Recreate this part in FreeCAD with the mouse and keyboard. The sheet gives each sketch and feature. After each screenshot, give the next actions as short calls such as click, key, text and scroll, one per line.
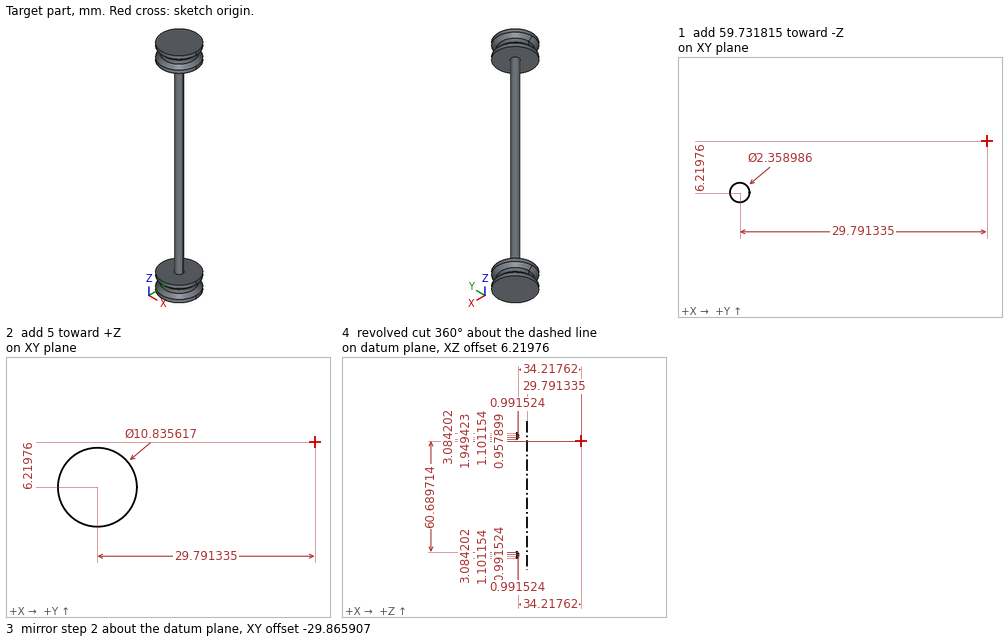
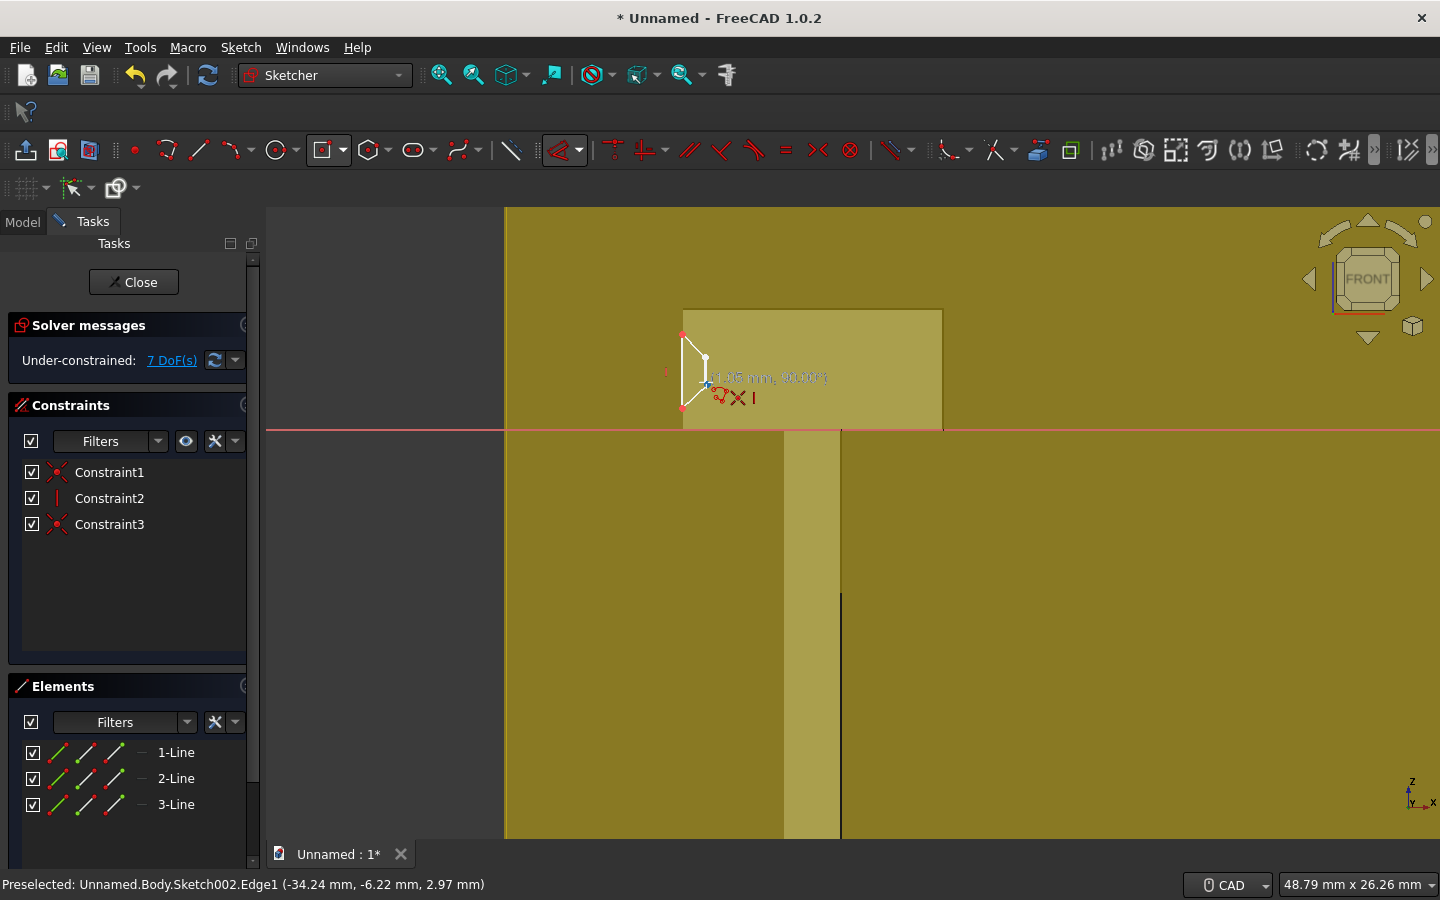
click(708, 385)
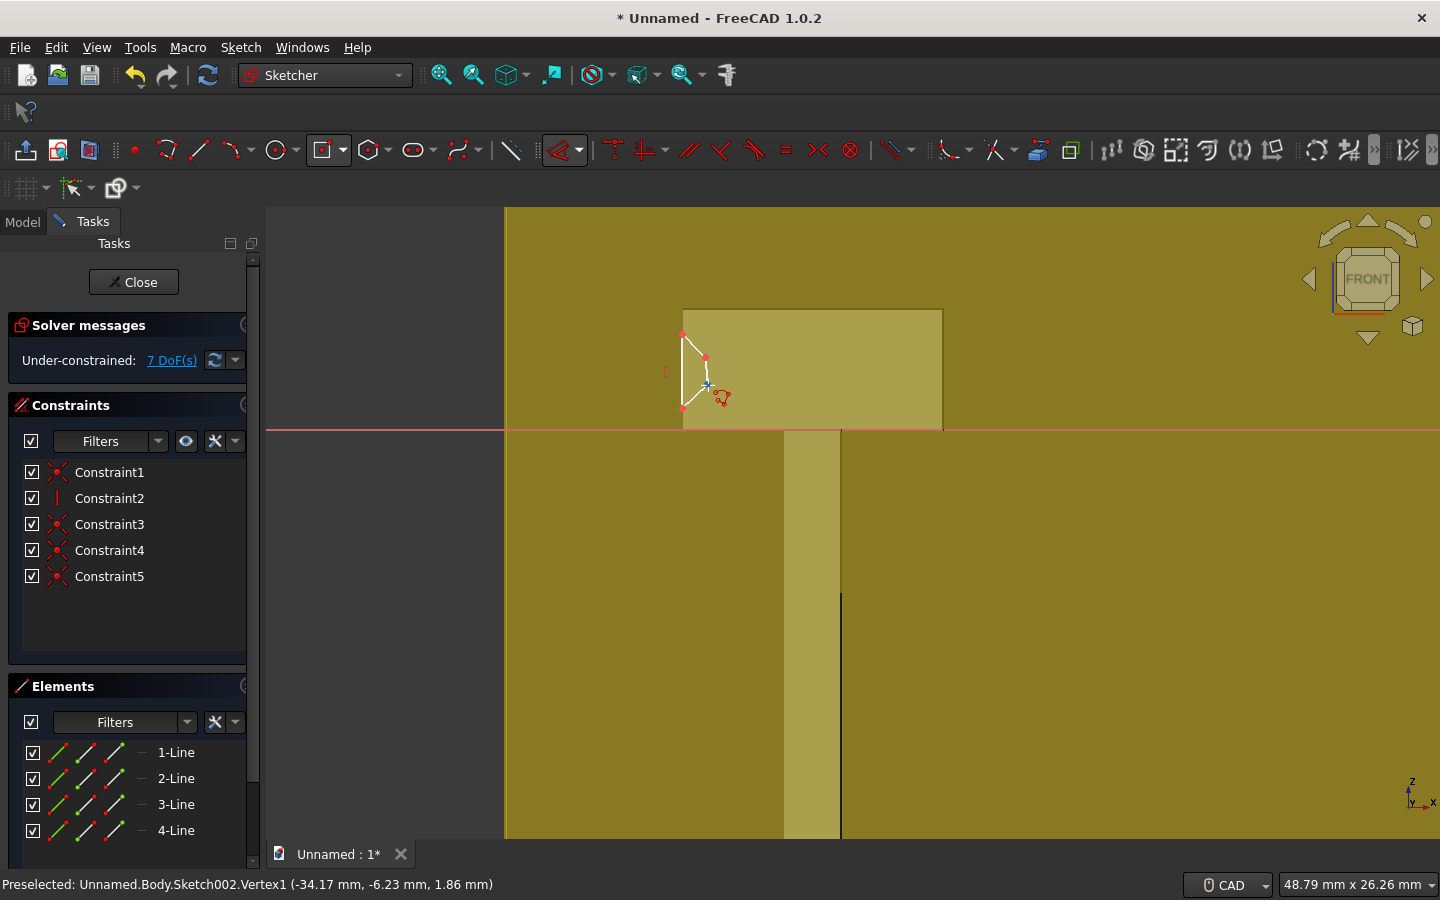
scroll(703, 365, down, 8)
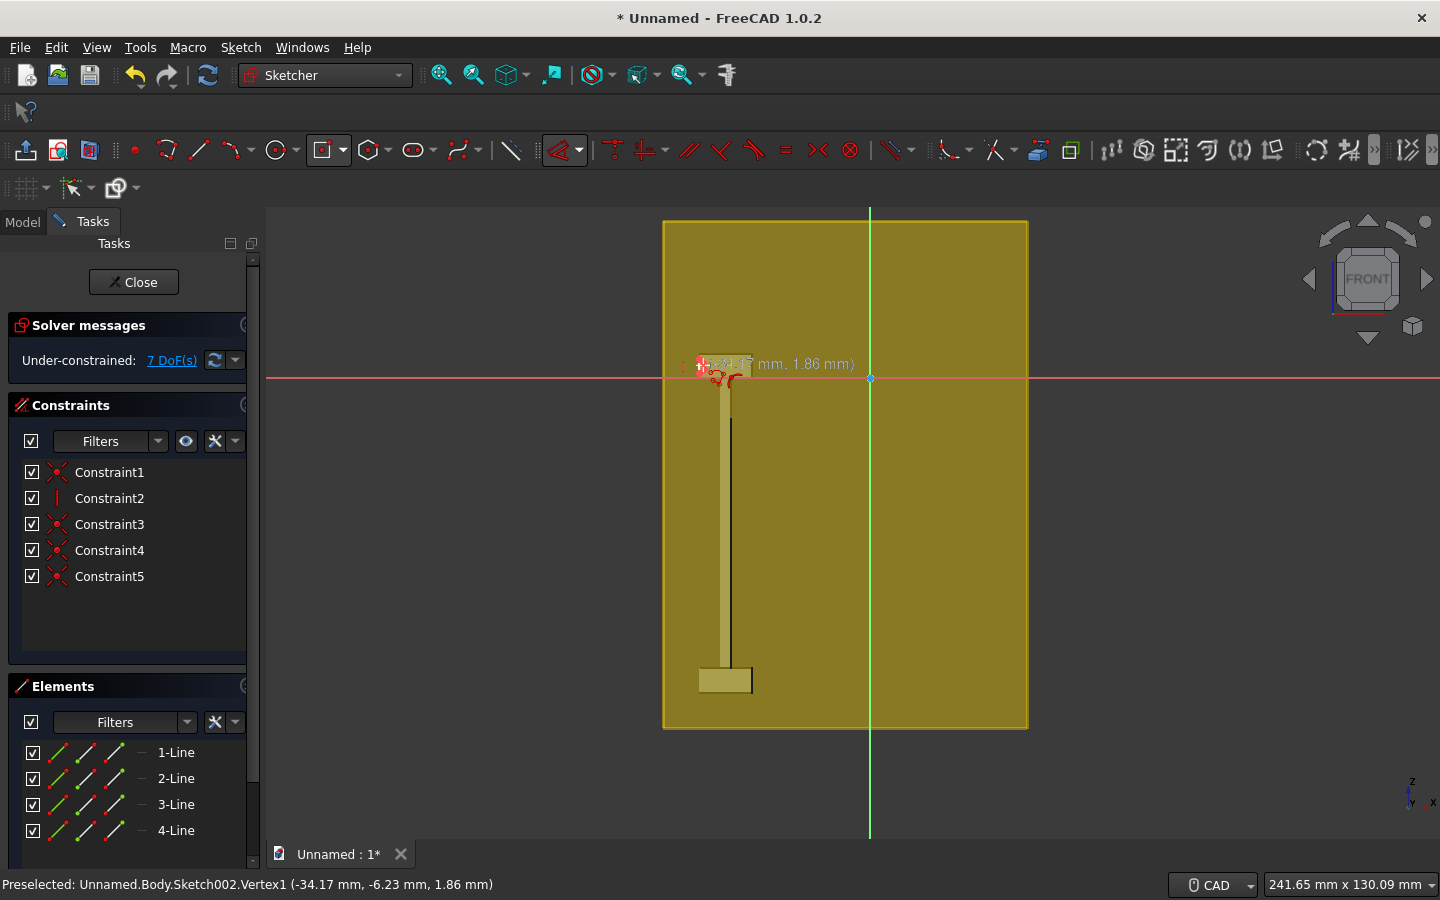
click(699, 673)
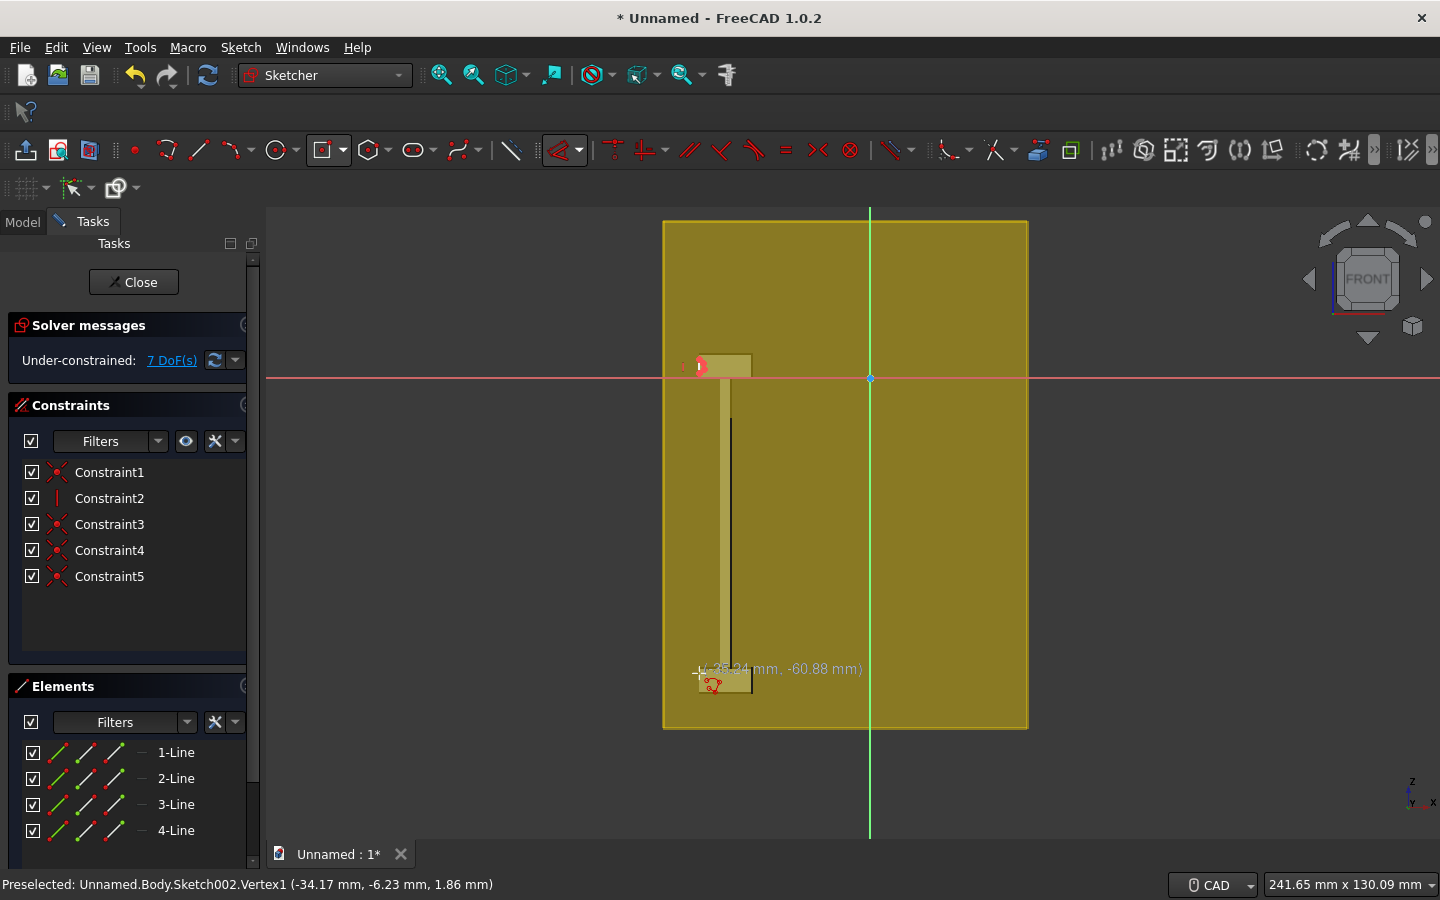
scroll(704, 678, up, 5)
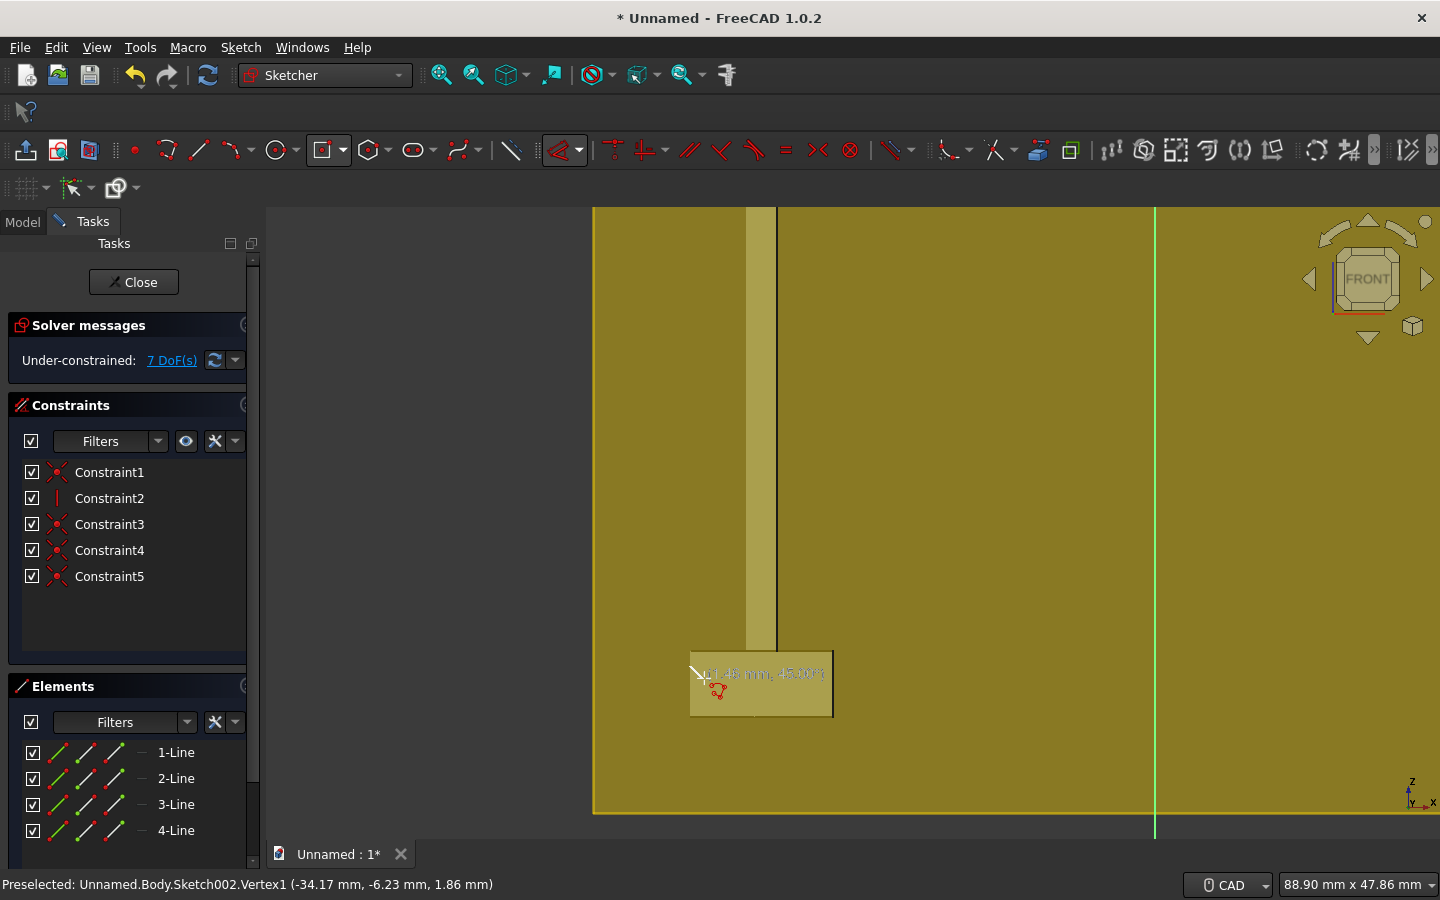
click(703, 676)
click(703, 691)
click(690, 704)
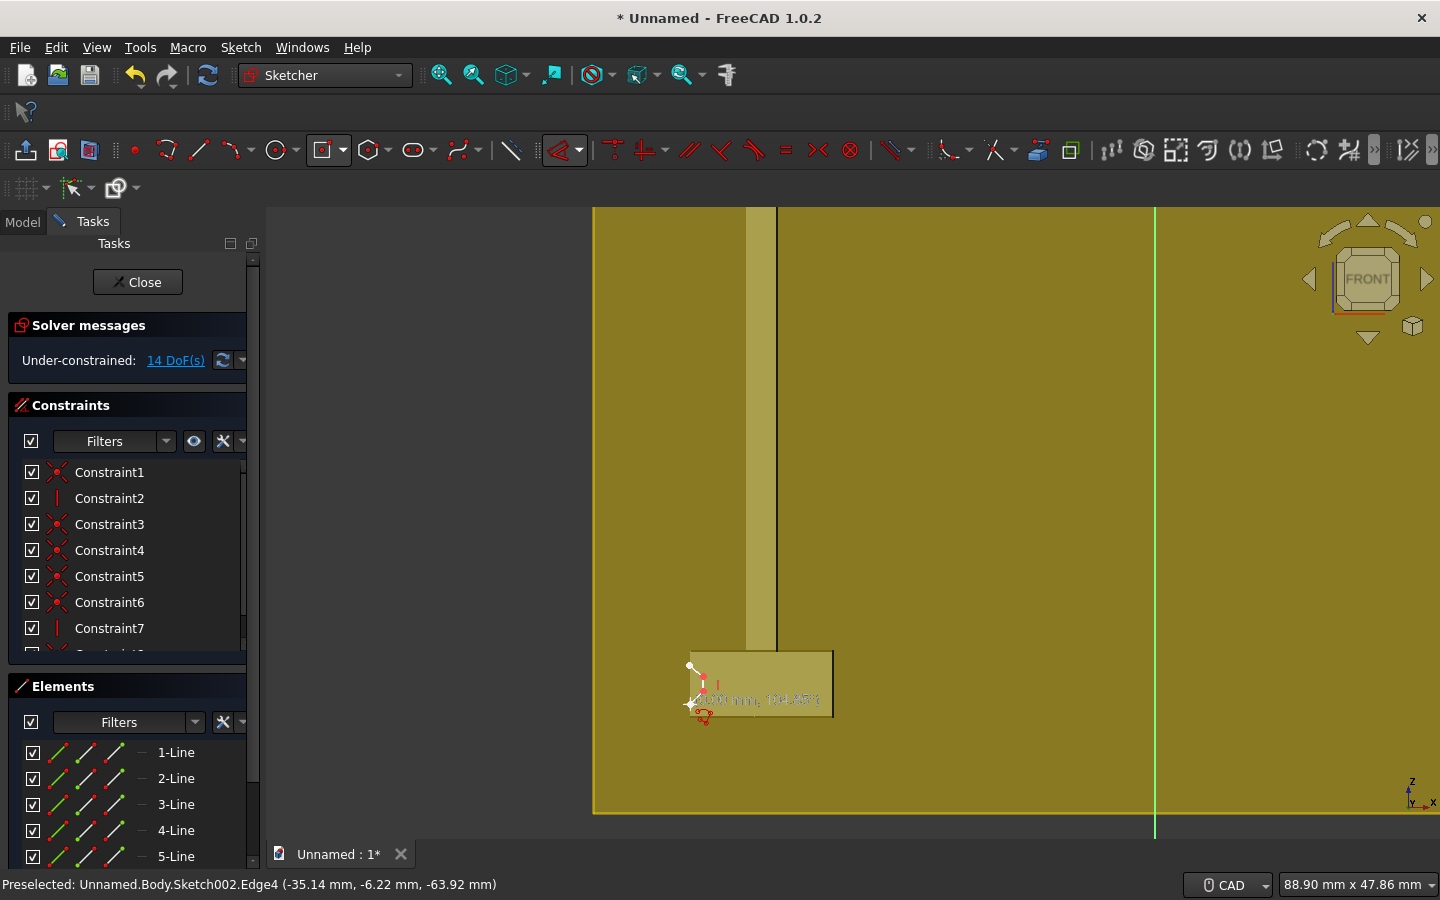
scroll(690, 663, up, 3)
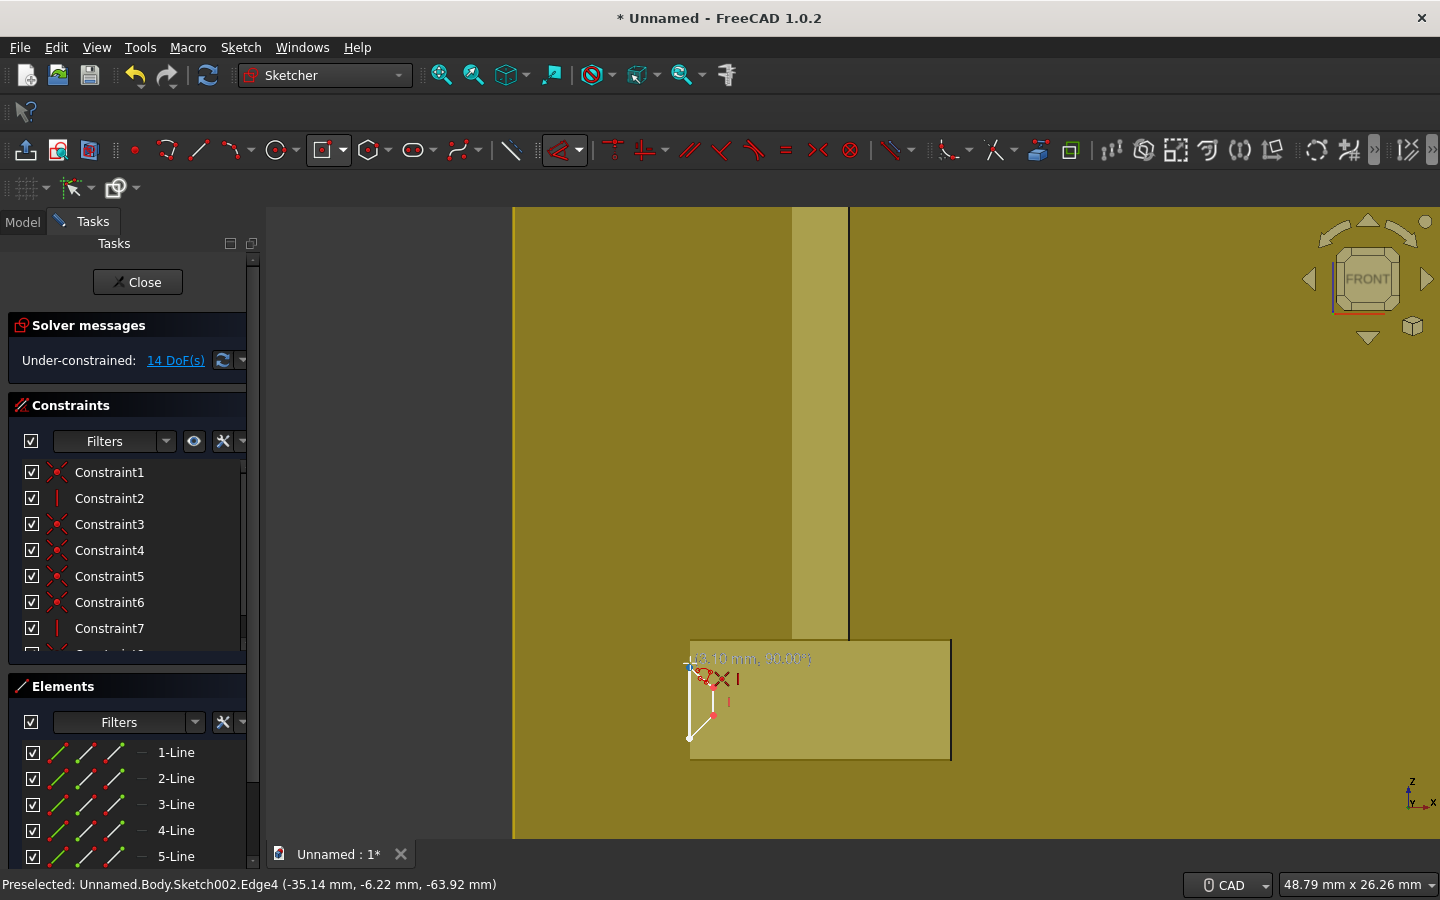
click(689, 668)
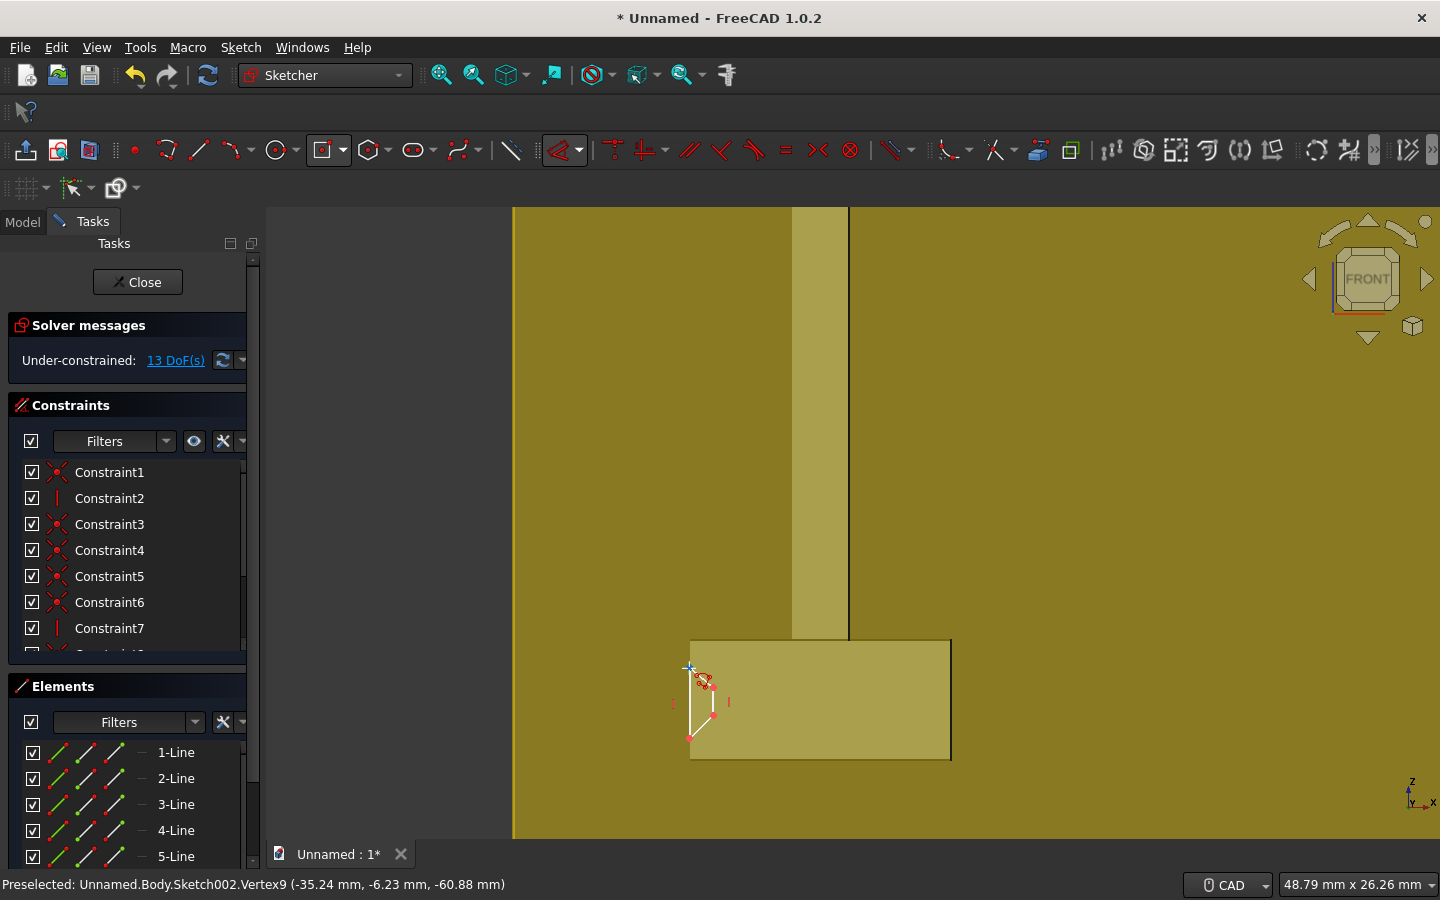
click(200, 150)